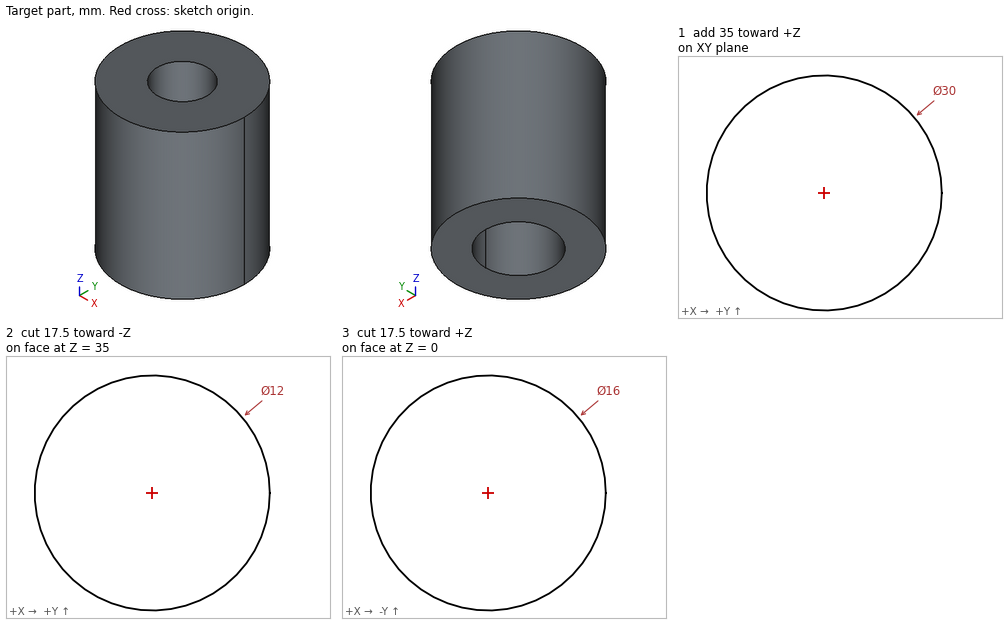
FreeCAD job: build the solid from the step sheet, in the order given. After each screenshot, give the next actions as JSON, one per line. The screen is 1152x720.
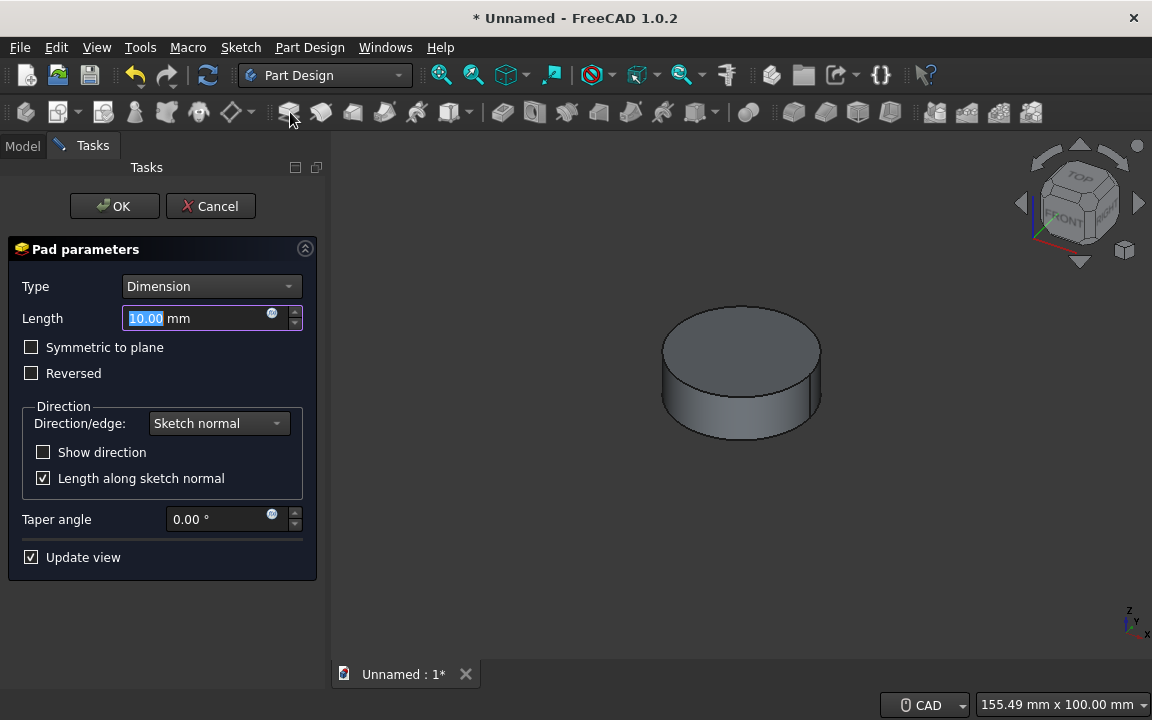
{"action": "type", "text": "35"}
{"action": "key", "text": "Tab"}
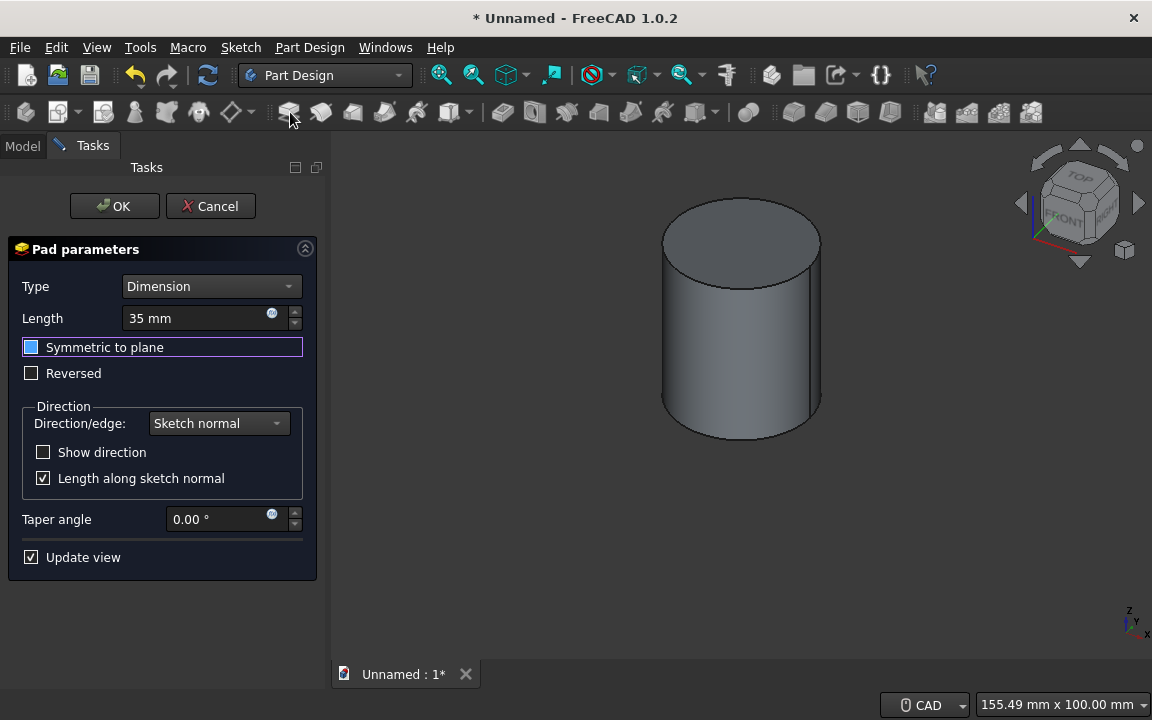
{"action": "left_click", "coordinate": [115, 206]}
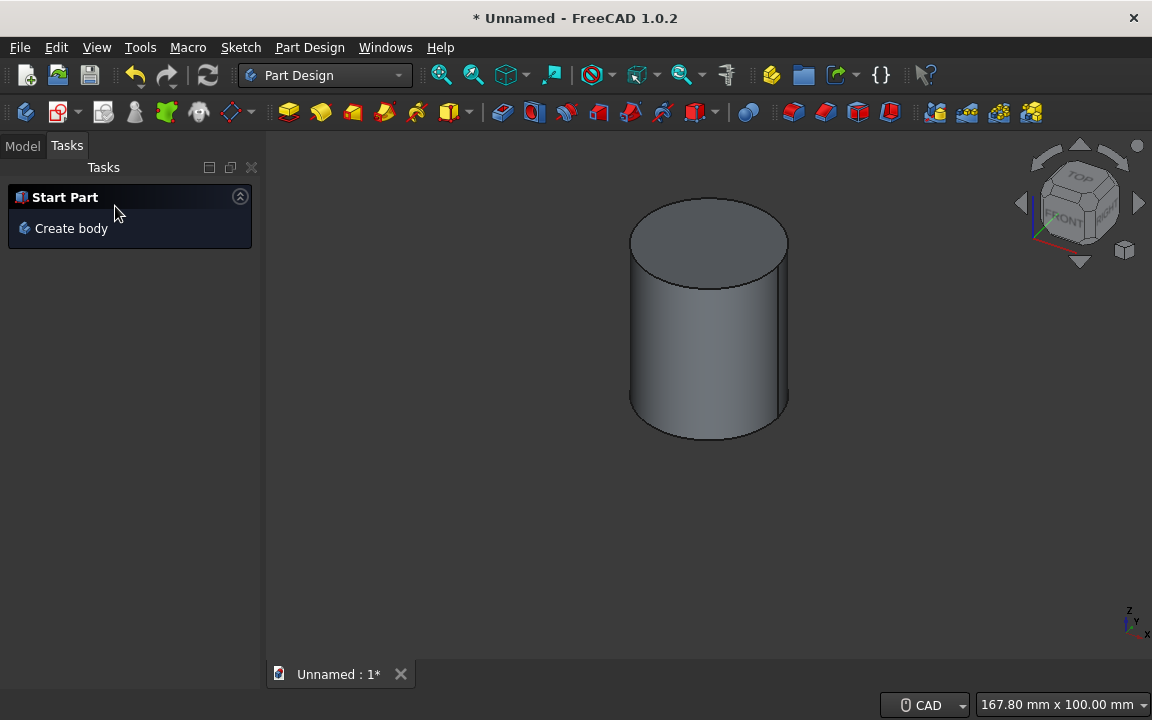
{"action": "left_click", "coordinate": [709, 243]}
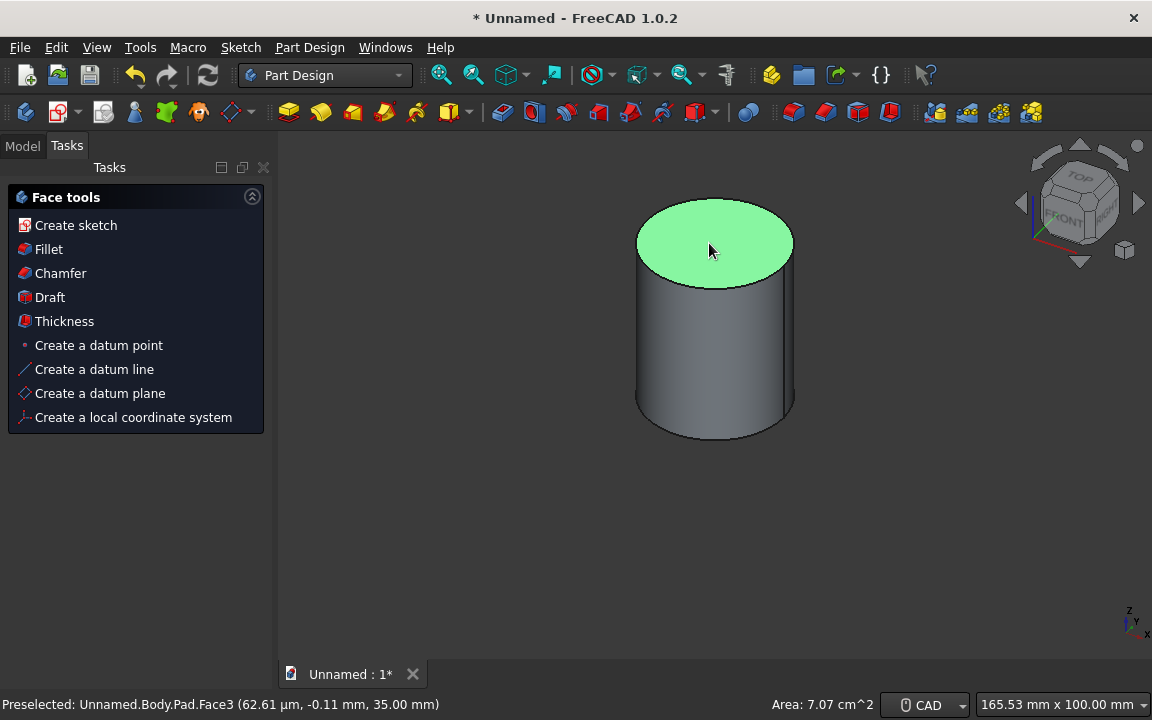
{"action": "left_click", "coordinate": [58, 112]}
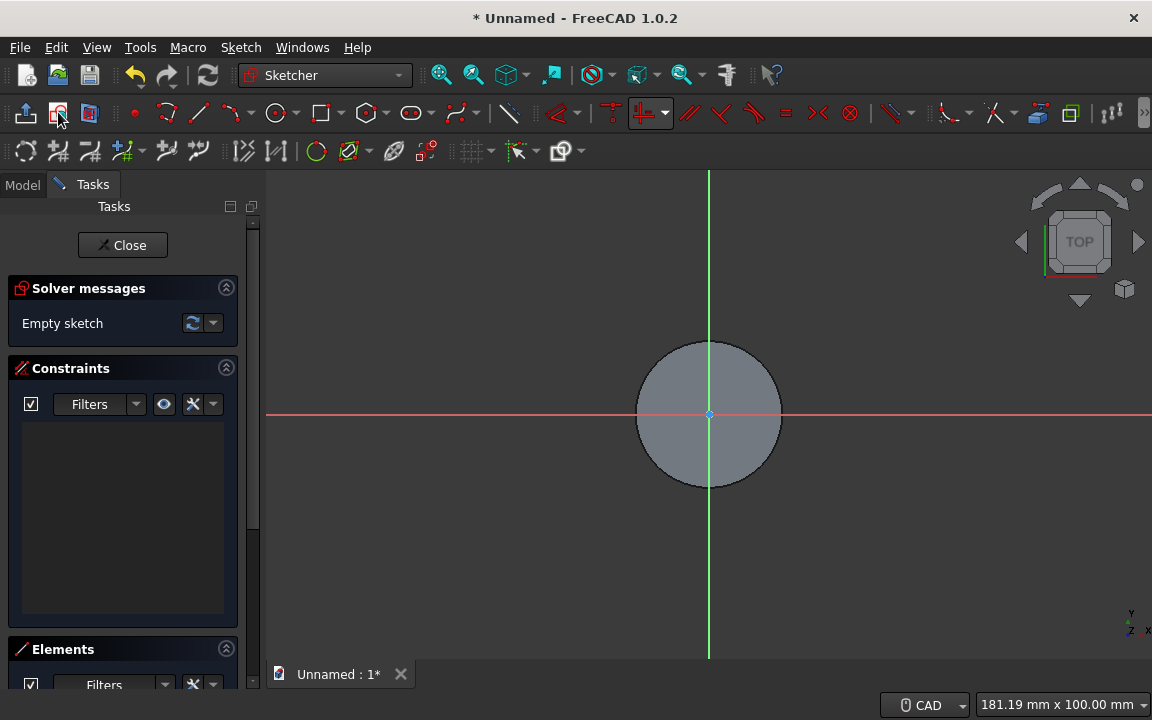
{"action": "scroll", "coordinate": [726, 414], "scroll_direction": "up", "scroll_amount": 8}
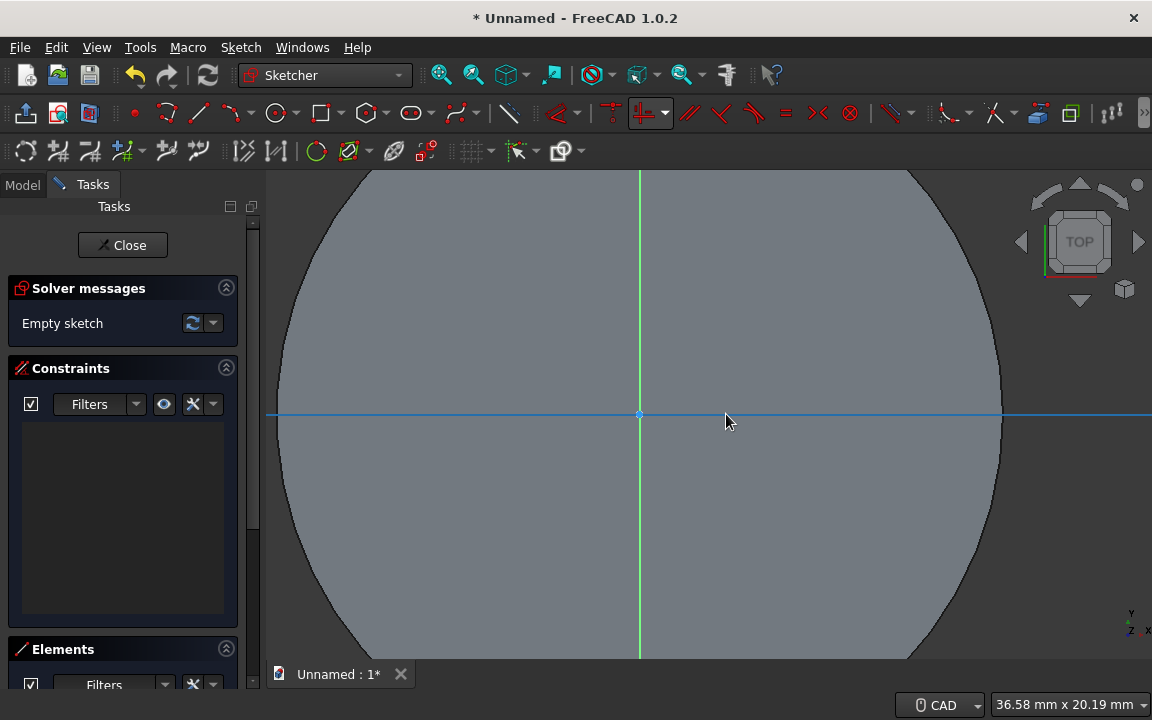
{"action": "key", "text": "g c"}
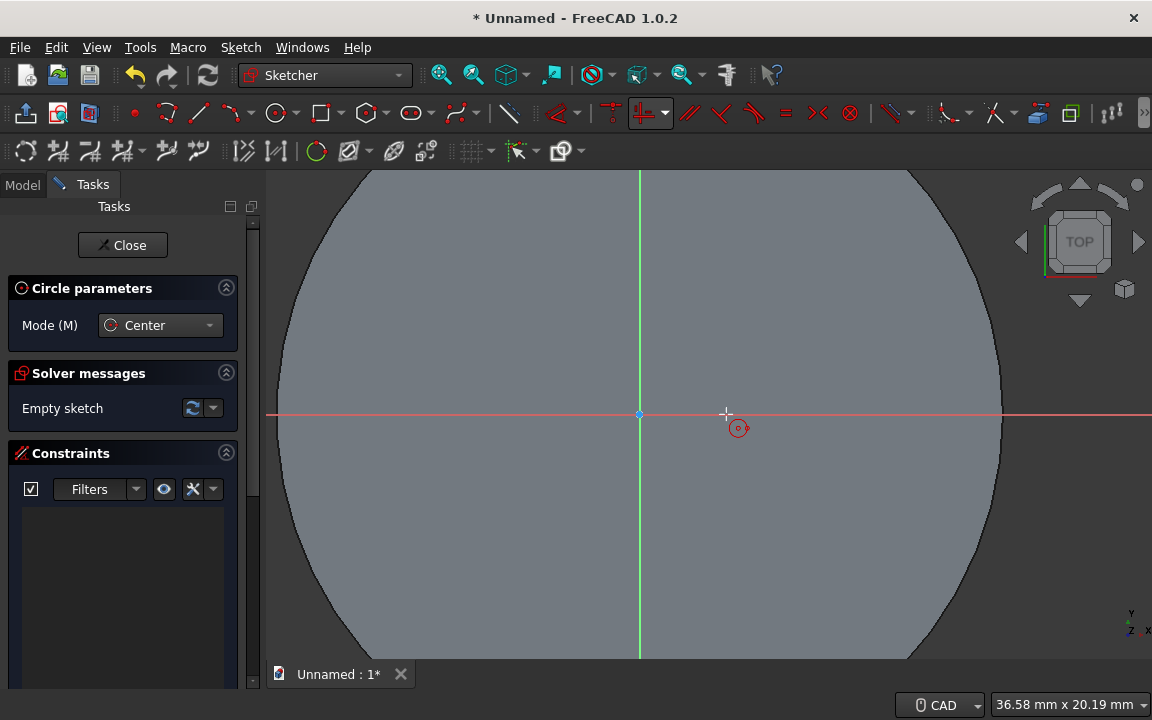
{"action": "left_click", "coordinate": [640, 414]}
{"action": "left_click", "coordinate": [743, 312]}
{"action": "key", "text": "Escape"}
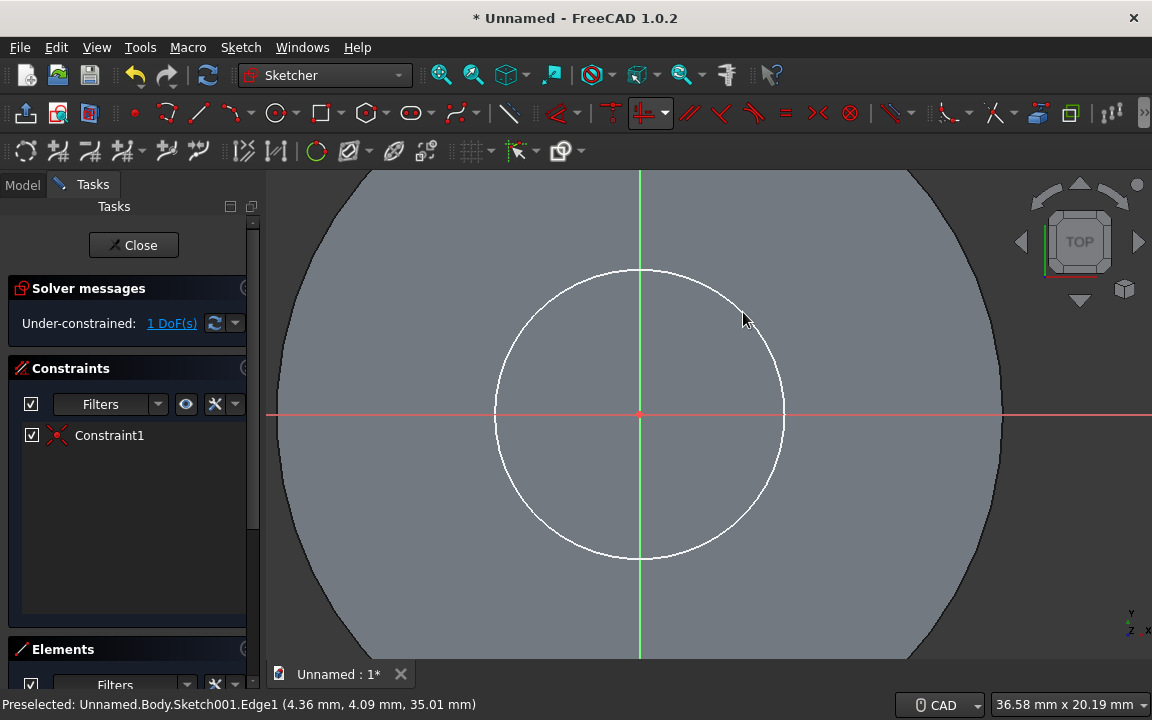
{"action": "key", "text": "d"}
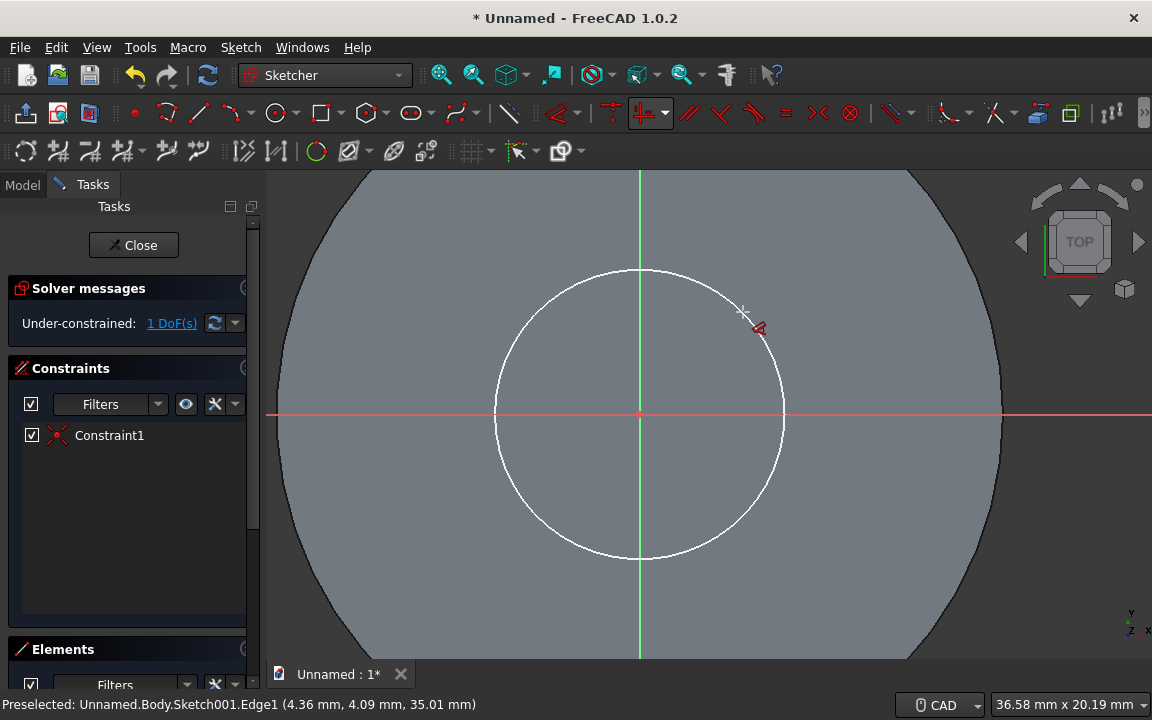
{"action": "left_click", "coordinate": [742, 312]}
{"action": "left_click", "coordinate": [765, 289]}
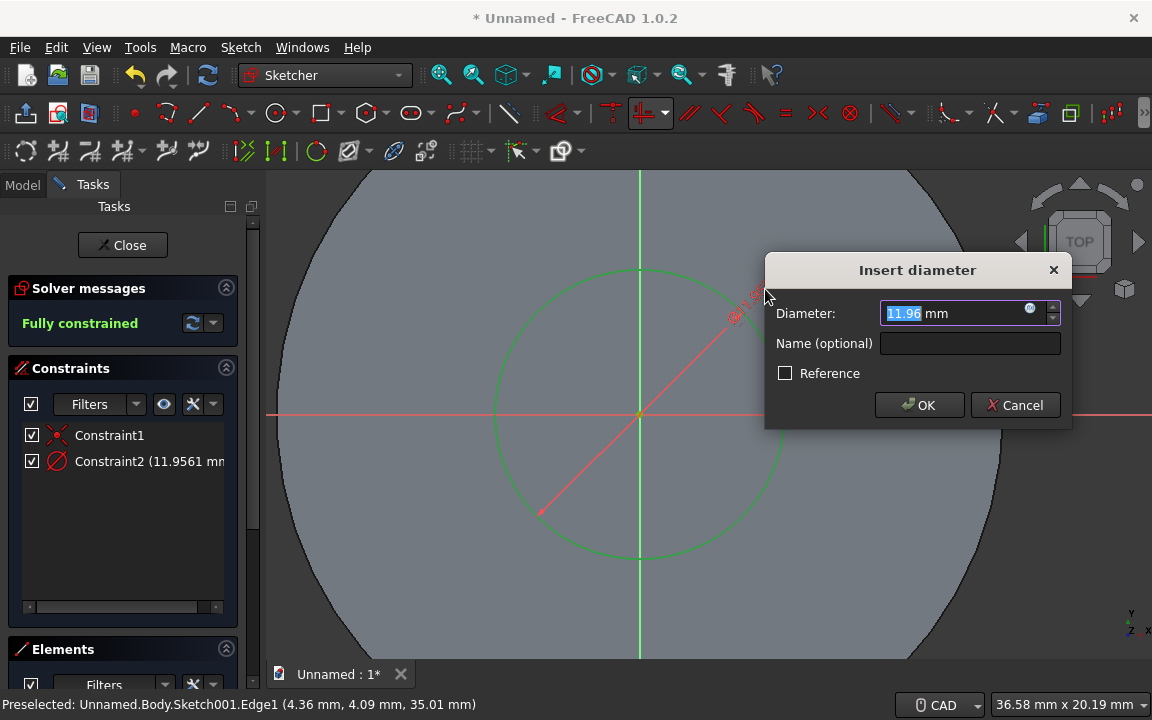
{"action": "type", "text": "12"}
{"action": "key", "text": "Return"}
{"action": "key", "text": "Escape"}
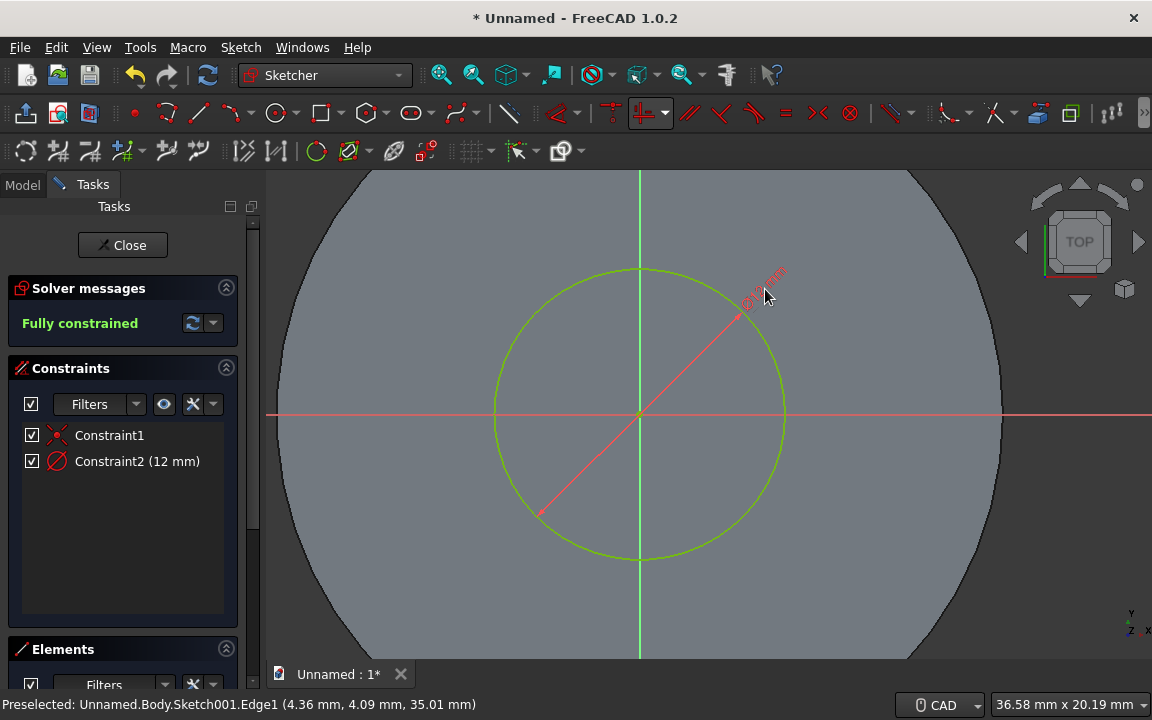
{"action": "left_click", "coordinate": [123, 245]}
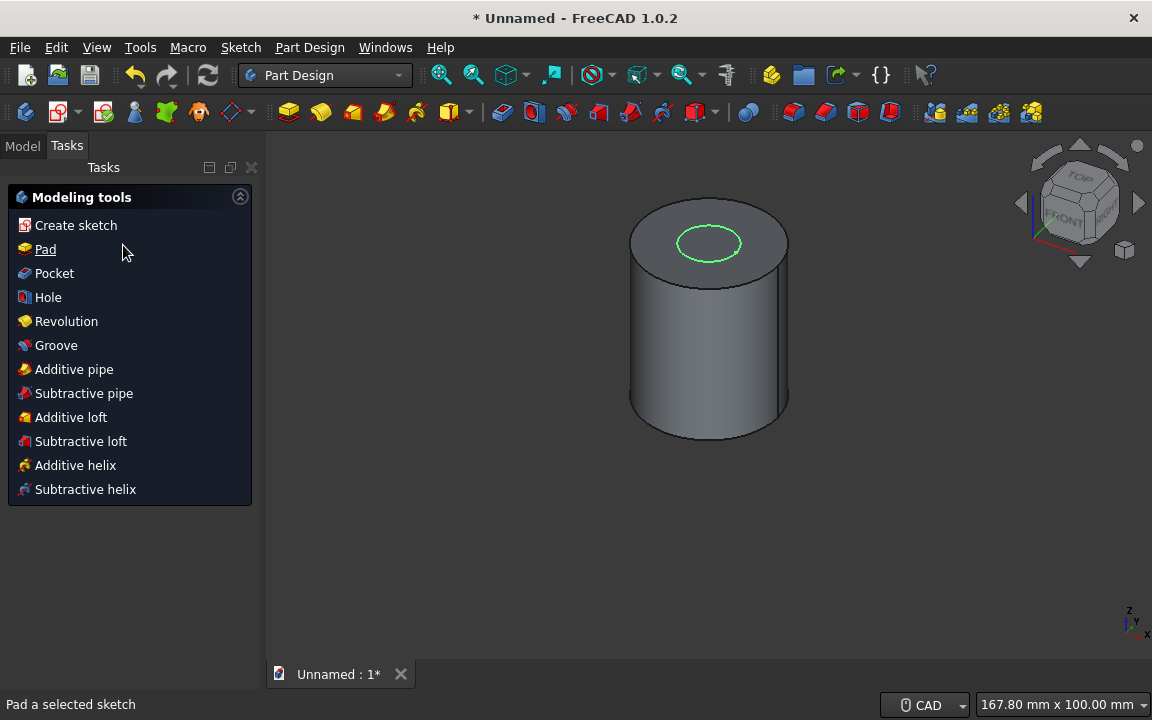
{"action": "left_click", "coordinate": [504, 112]}